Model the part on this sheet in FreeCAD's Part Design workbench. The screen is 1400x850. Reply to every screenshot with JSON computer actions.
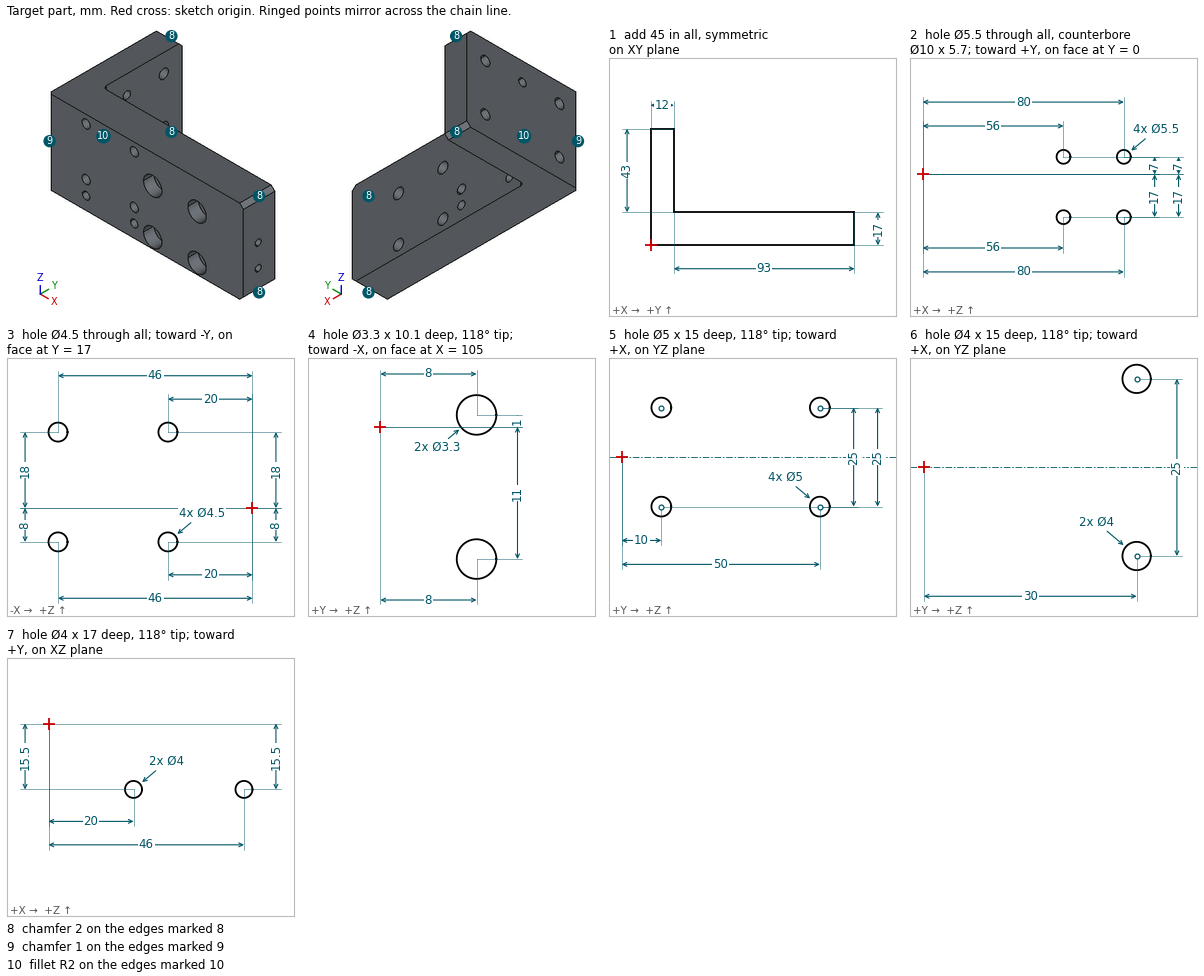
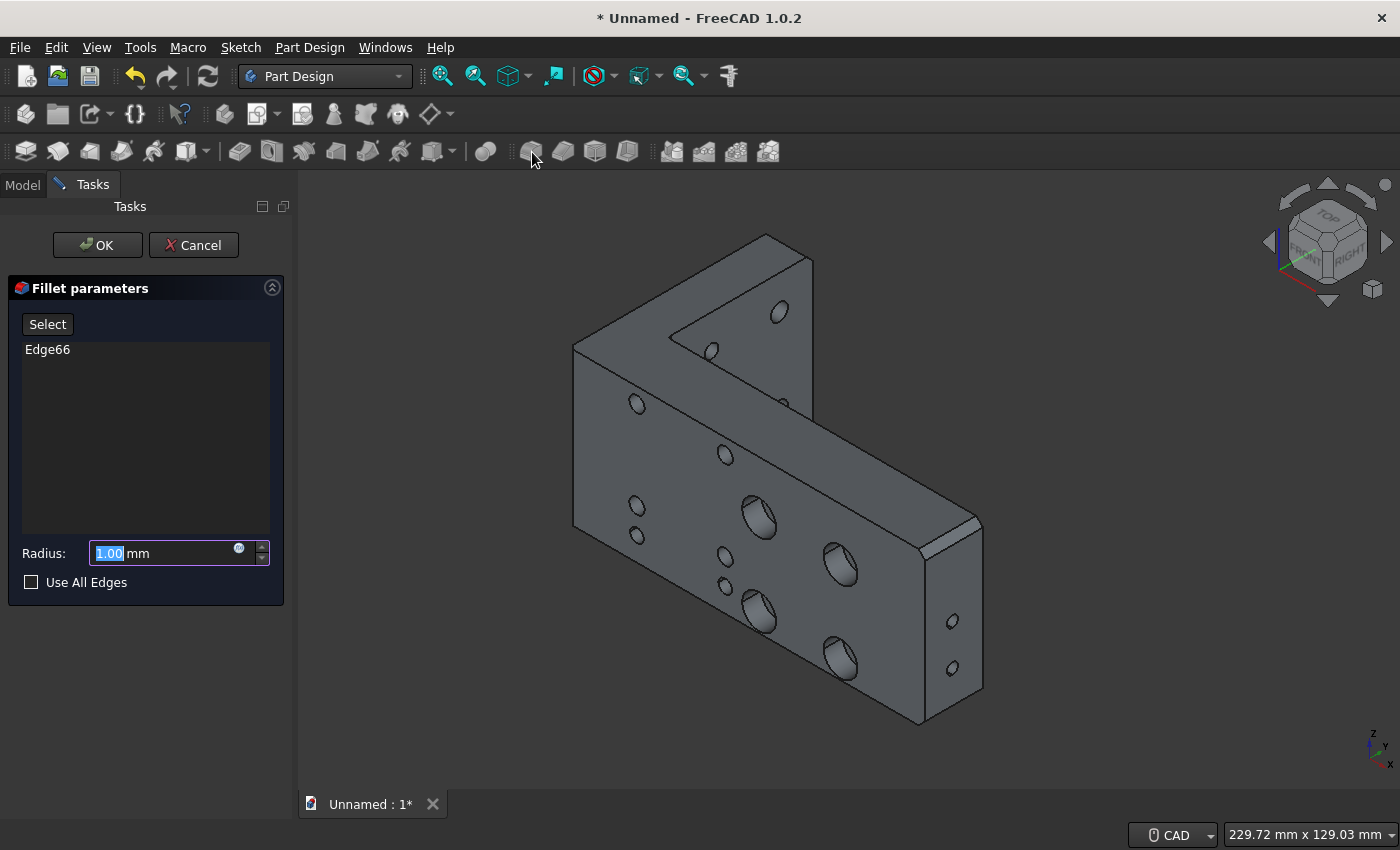
{"action": "type", "text": "2"}
{"action": "key", "text": "Tab"}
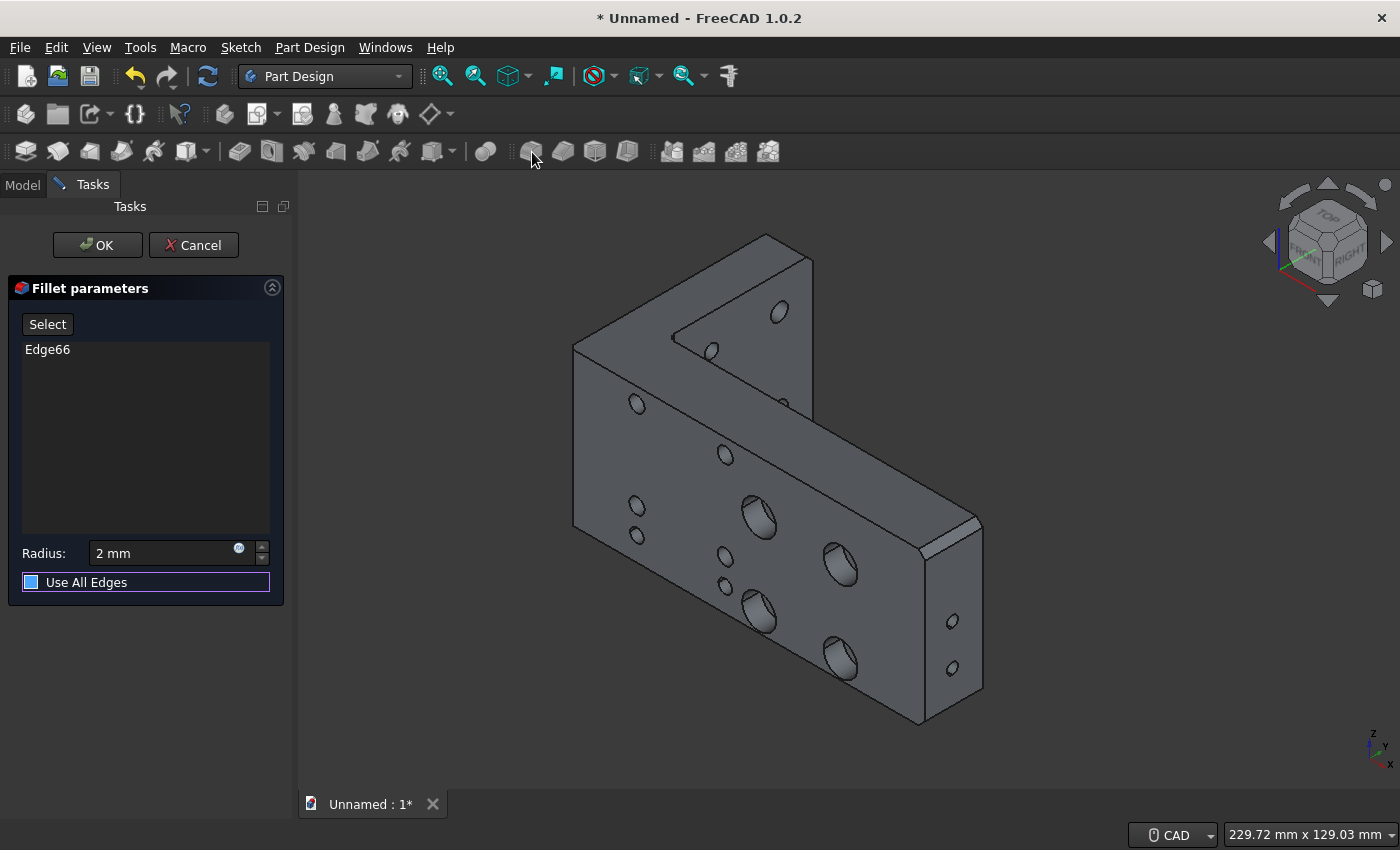
{"action": "left_click", "coordinate": [98, 245]}